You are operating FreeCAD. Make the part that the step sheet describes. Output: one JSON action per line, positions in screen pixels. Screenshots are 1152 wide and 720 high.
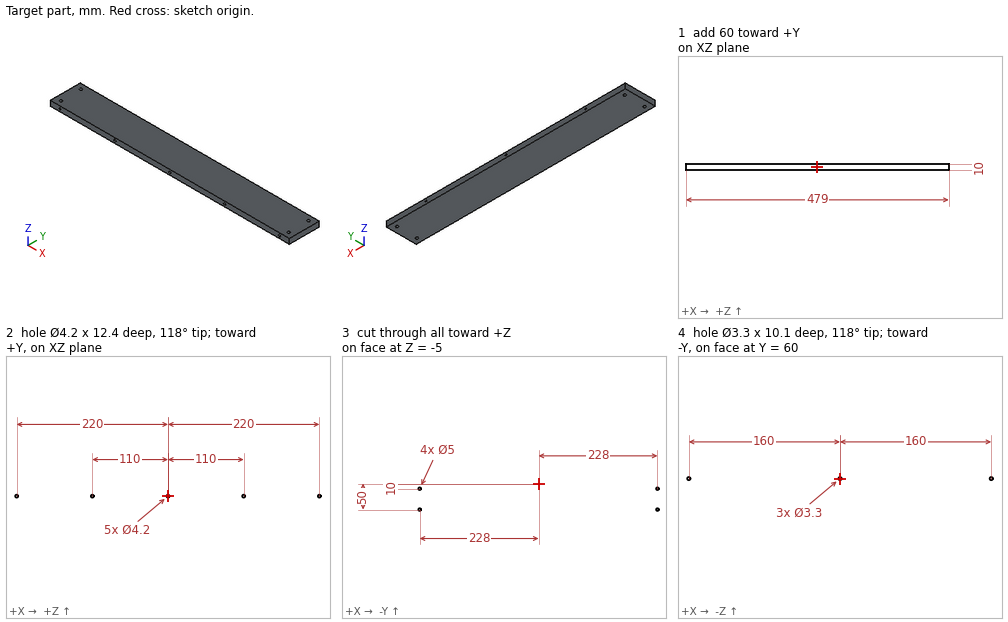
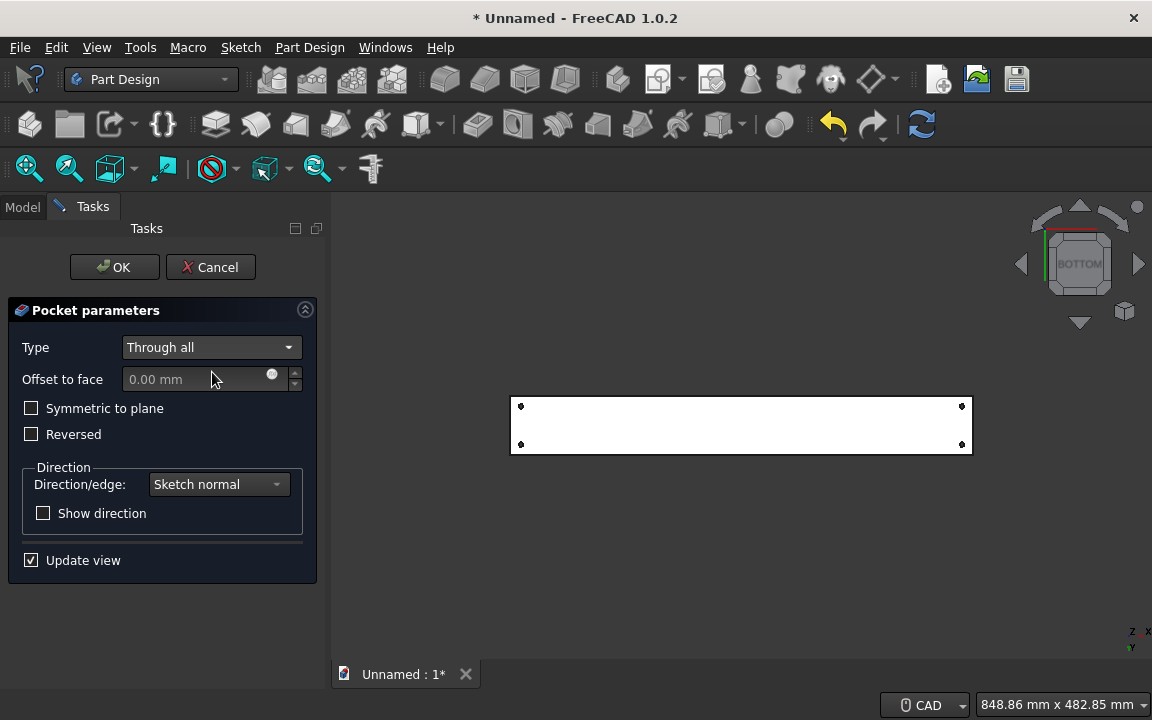
{"action": "left_click", "coordinate": [115, 267]}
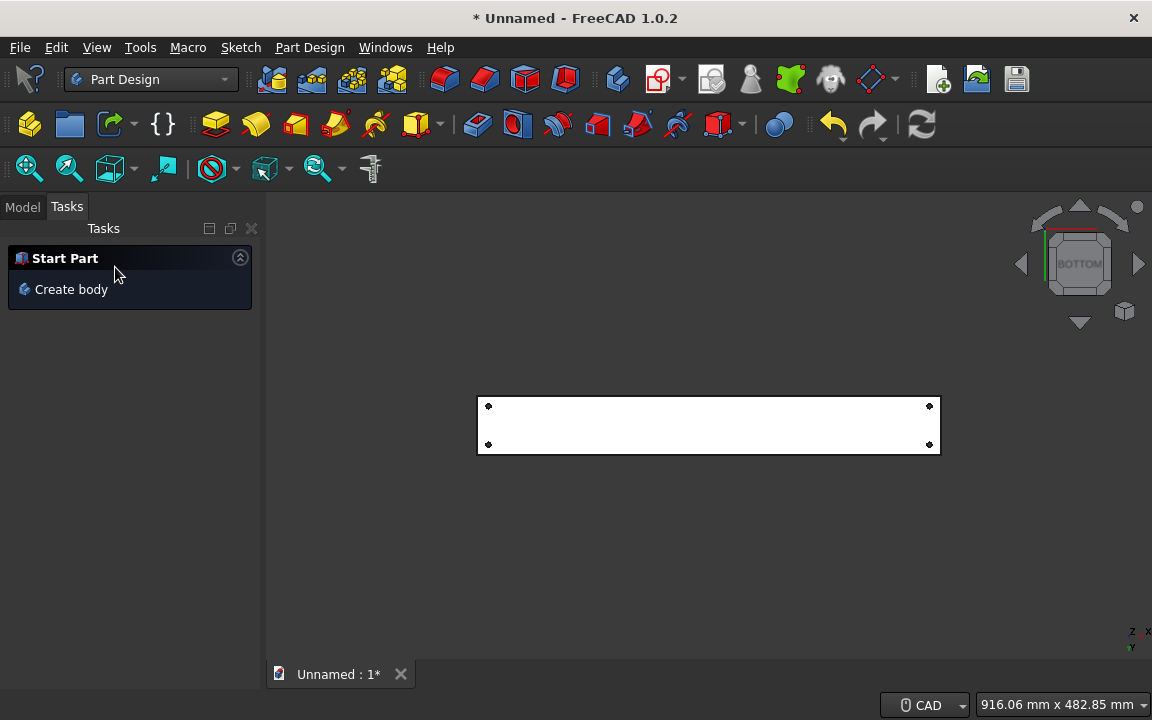
{"action": "key", "text": "4"}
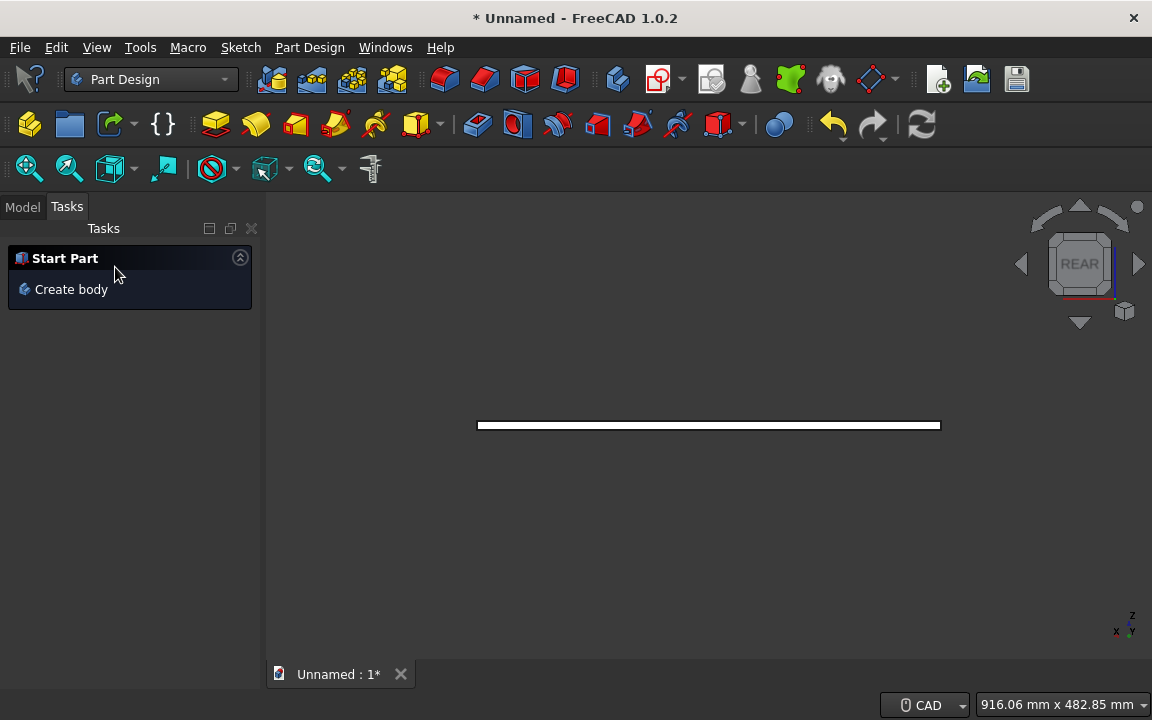
{"action": "scroll", "coordinate": [510, 424], "scroll_direction": "up", "scroll_amount": 5}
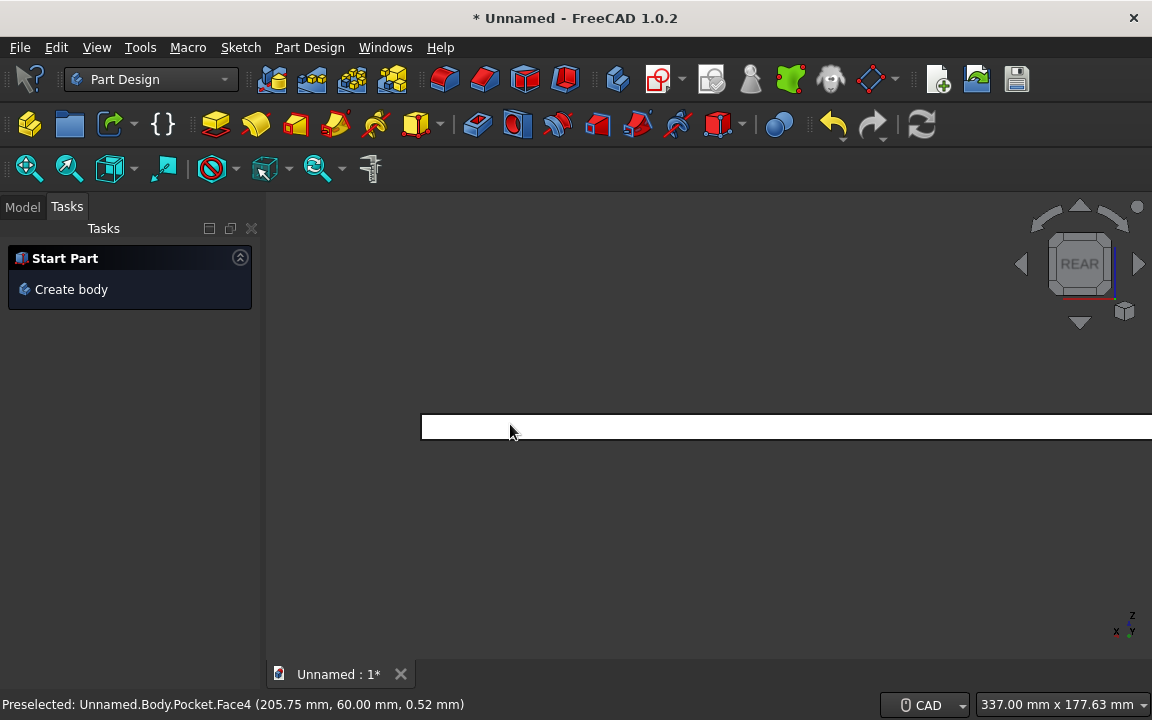
{"action": "left_click", "coordinate": [511, 426]}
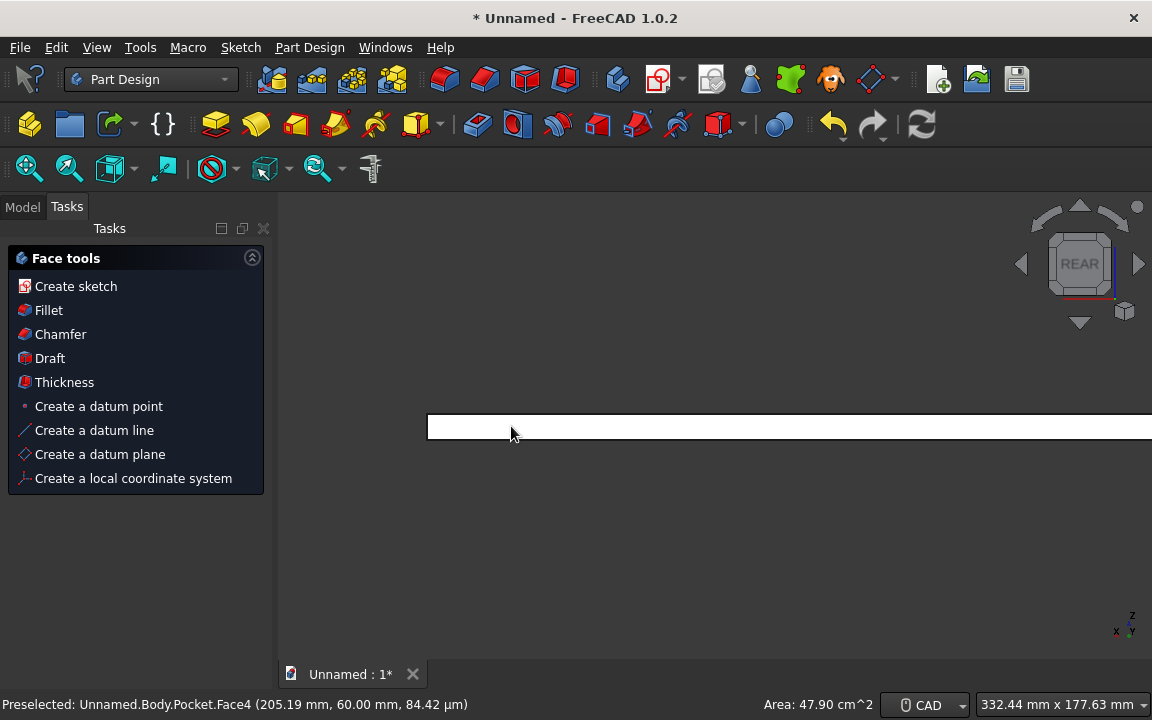
{"action": "left_click", "coordinate": [658, 80]}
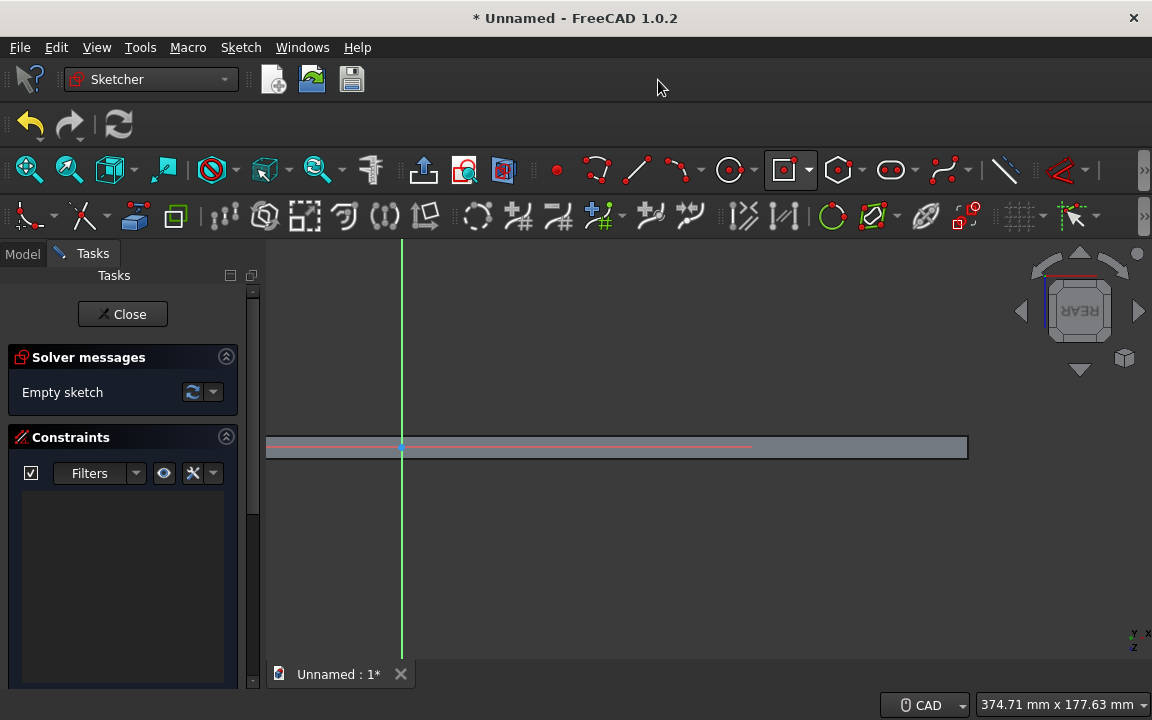
{"action": "scroll", "coordinate": [987, 452], "scroll_direction": "down", "scroll_amount": 2}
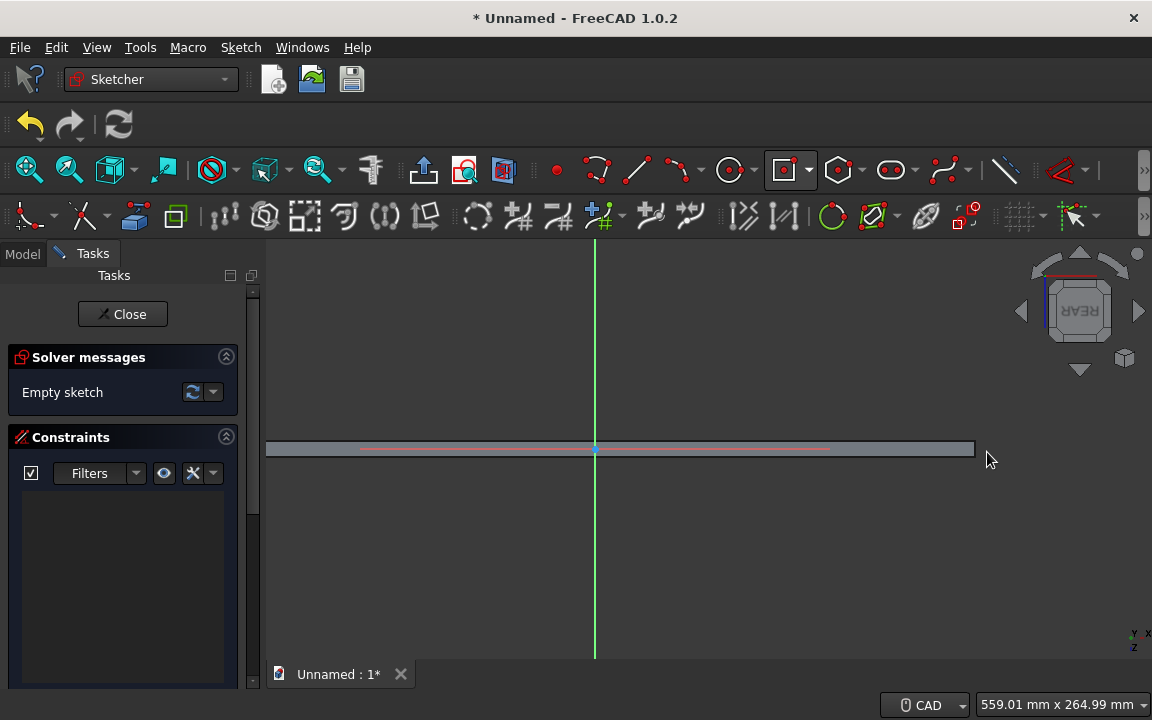
{"action": "left_click", "coordinate": [730, 170]}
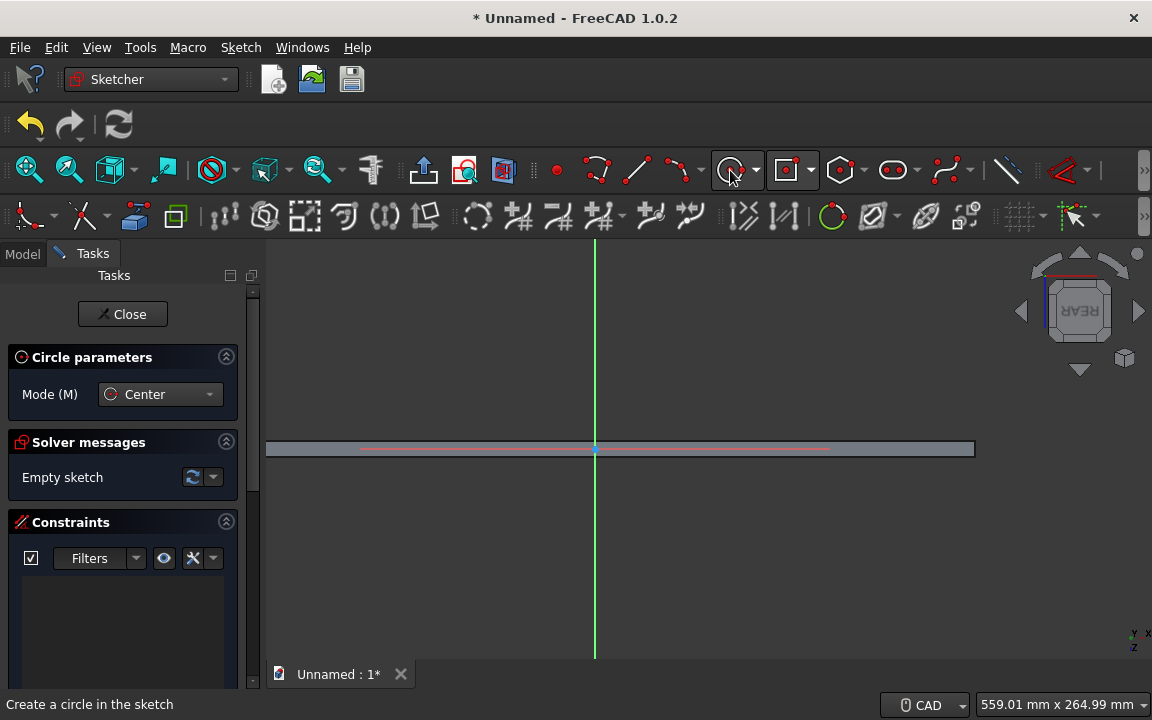
{"action": "scroll", "coordinate": [595, 449], "scroll_direction": "up", "scroll_amount": 11}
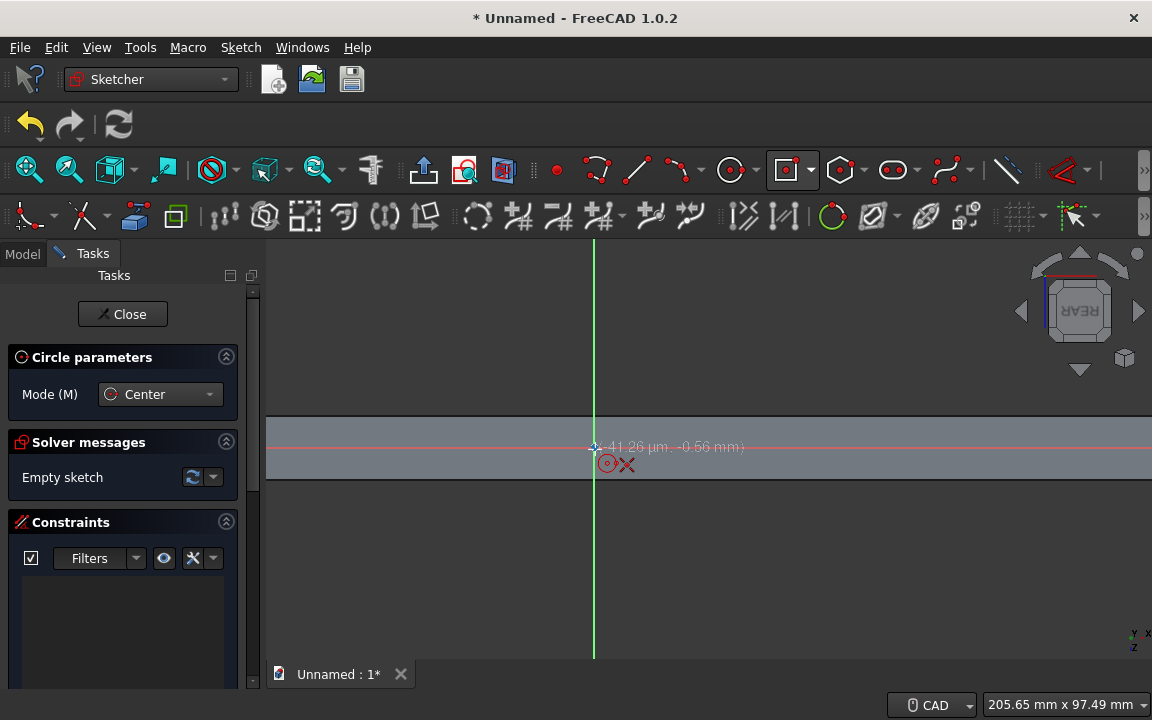
{"action": "scroll", "coordinate": [646, 449], "scroll_direction": "down", "scroll_amount": 11}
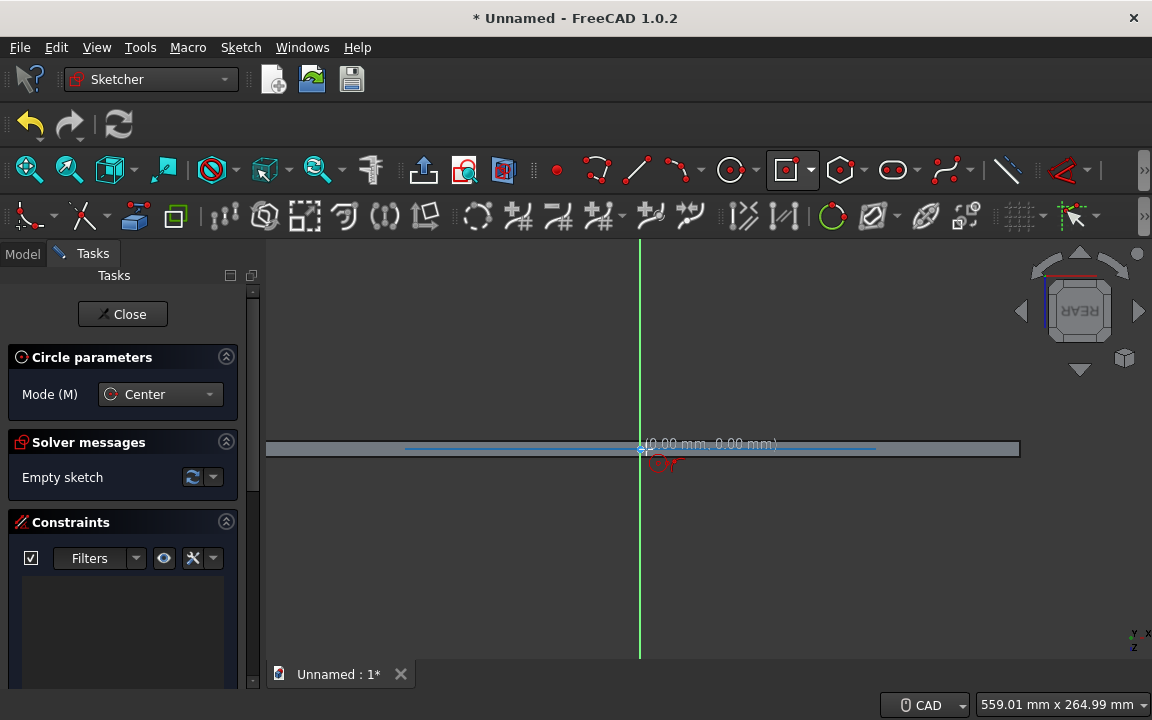
{"action": "left_click", "coordinate": [640, 449]}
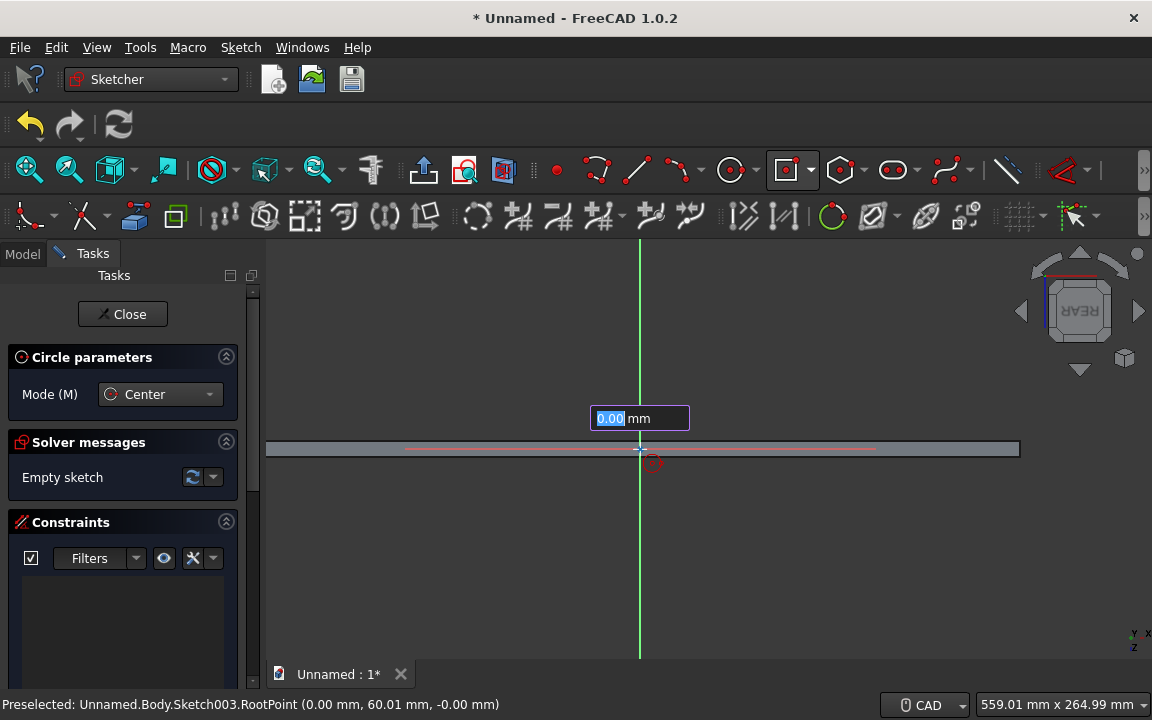
{"action": "scroll", "coordinate": [642, 447], "scroll_direction": "up", "scroll_amount": 11}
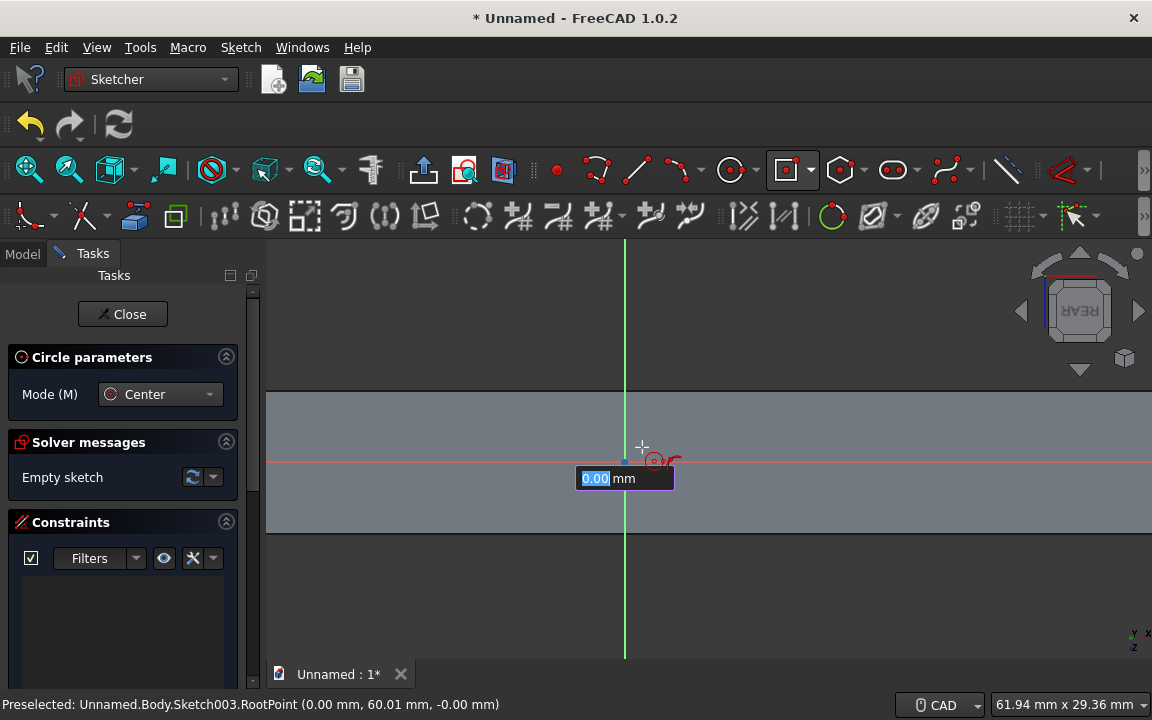
{"action": "left_click", "coordinate": [641, 445]}